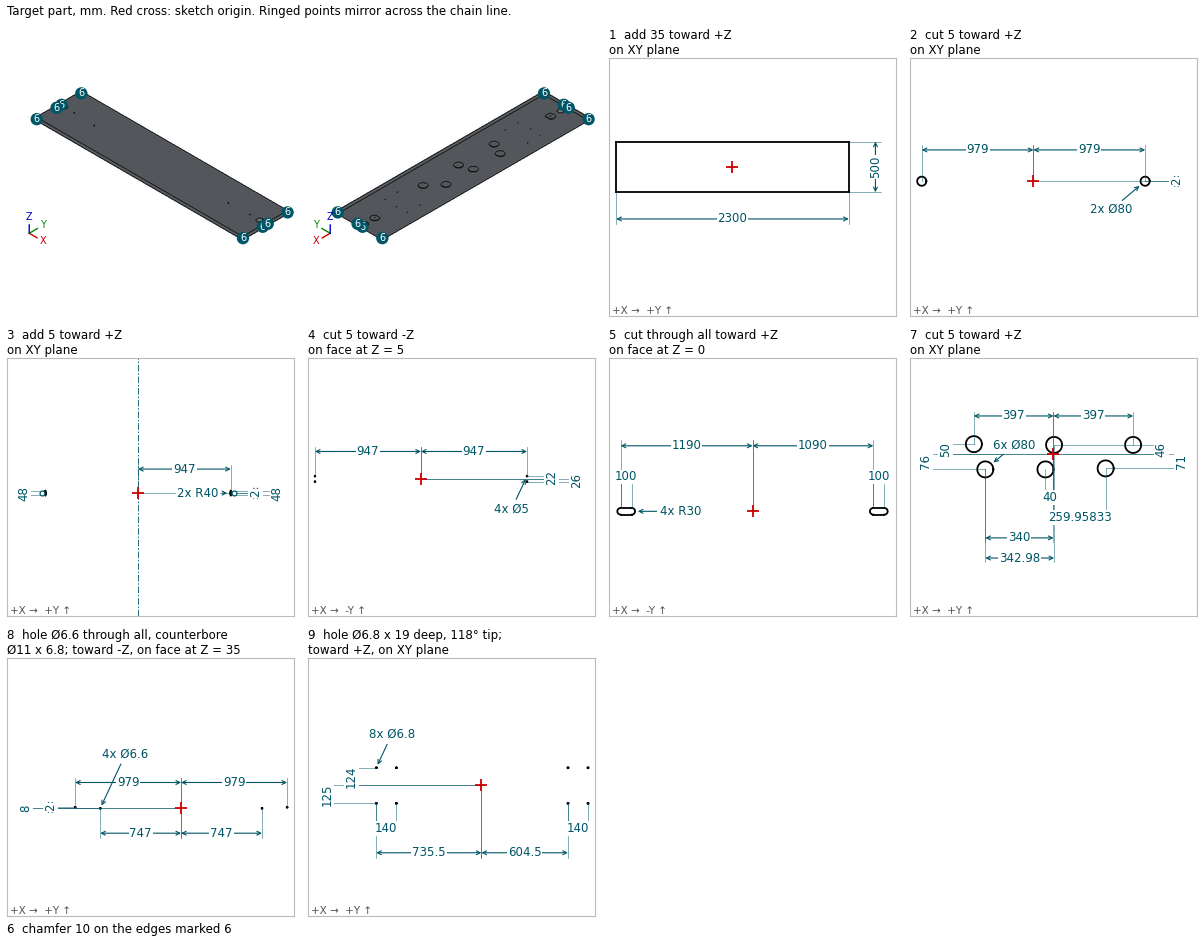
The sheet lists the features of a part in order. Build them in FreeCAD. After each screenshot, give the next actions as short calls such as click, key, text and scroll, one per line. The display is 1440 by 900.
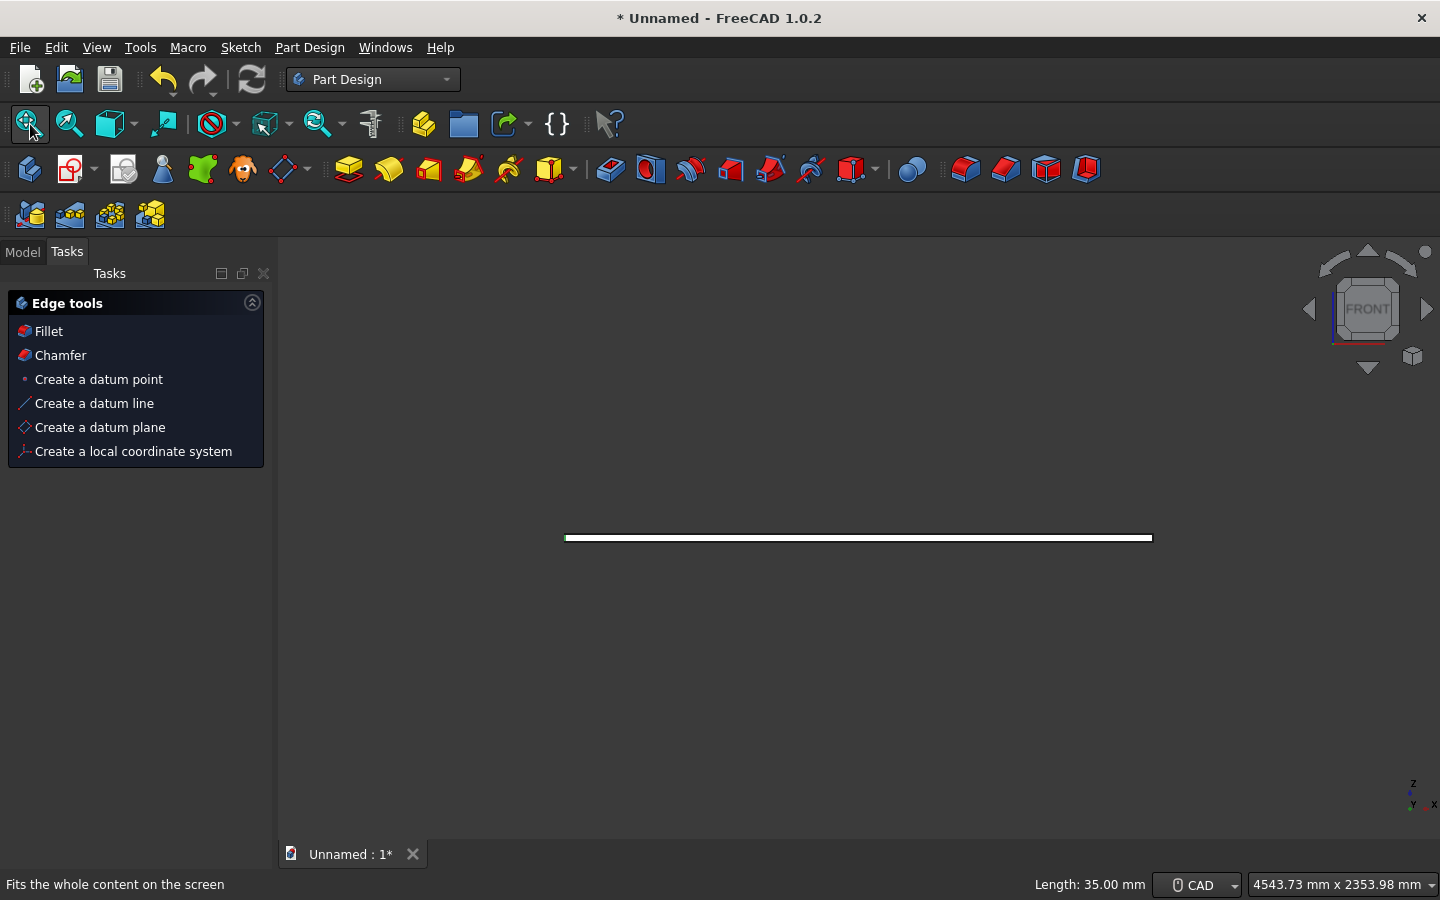
key(3)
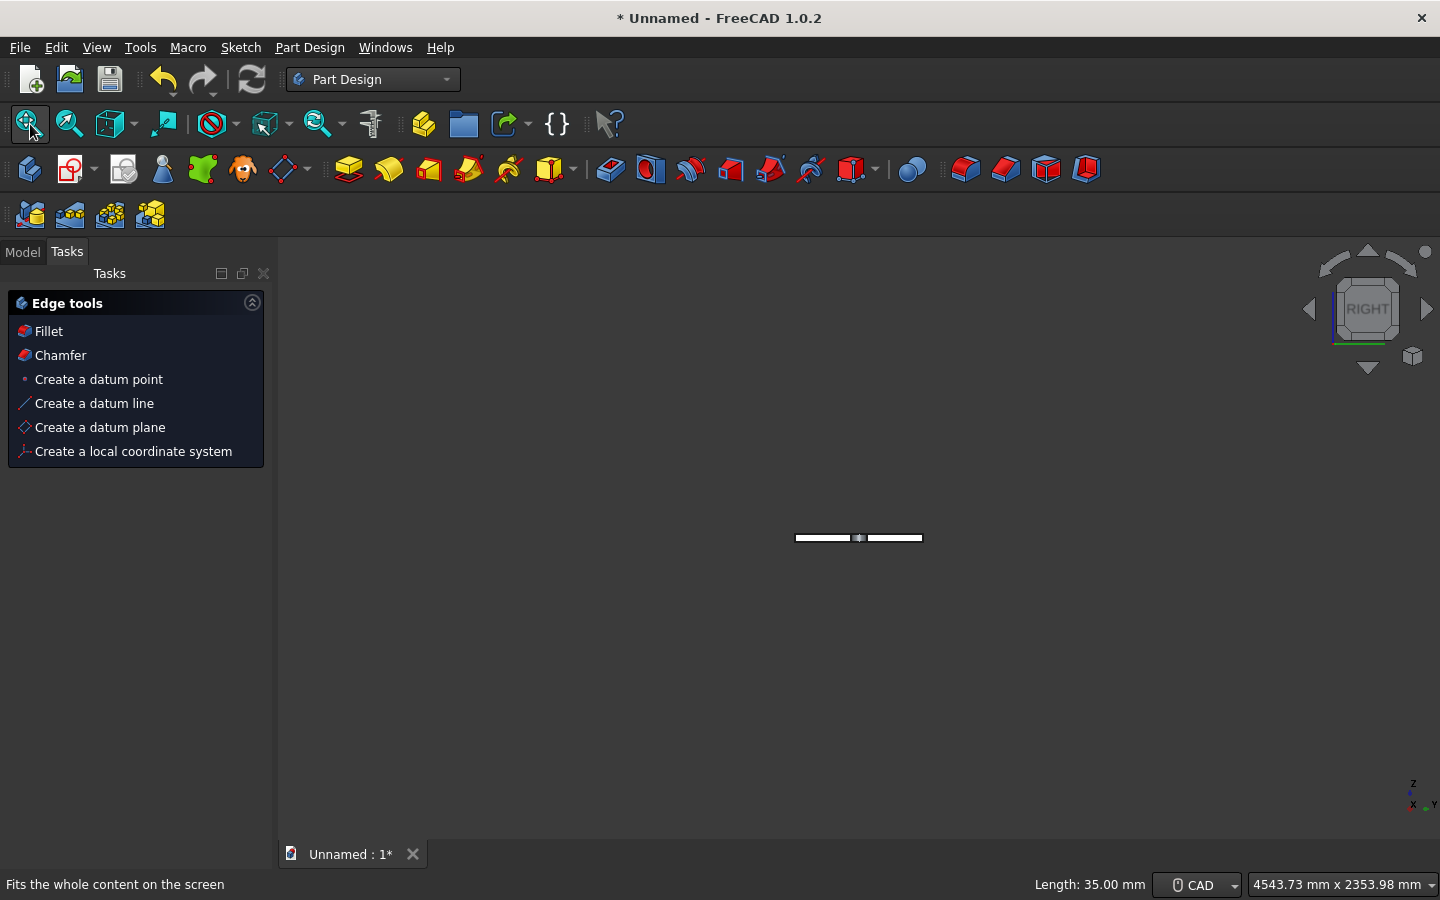
click(30, 124)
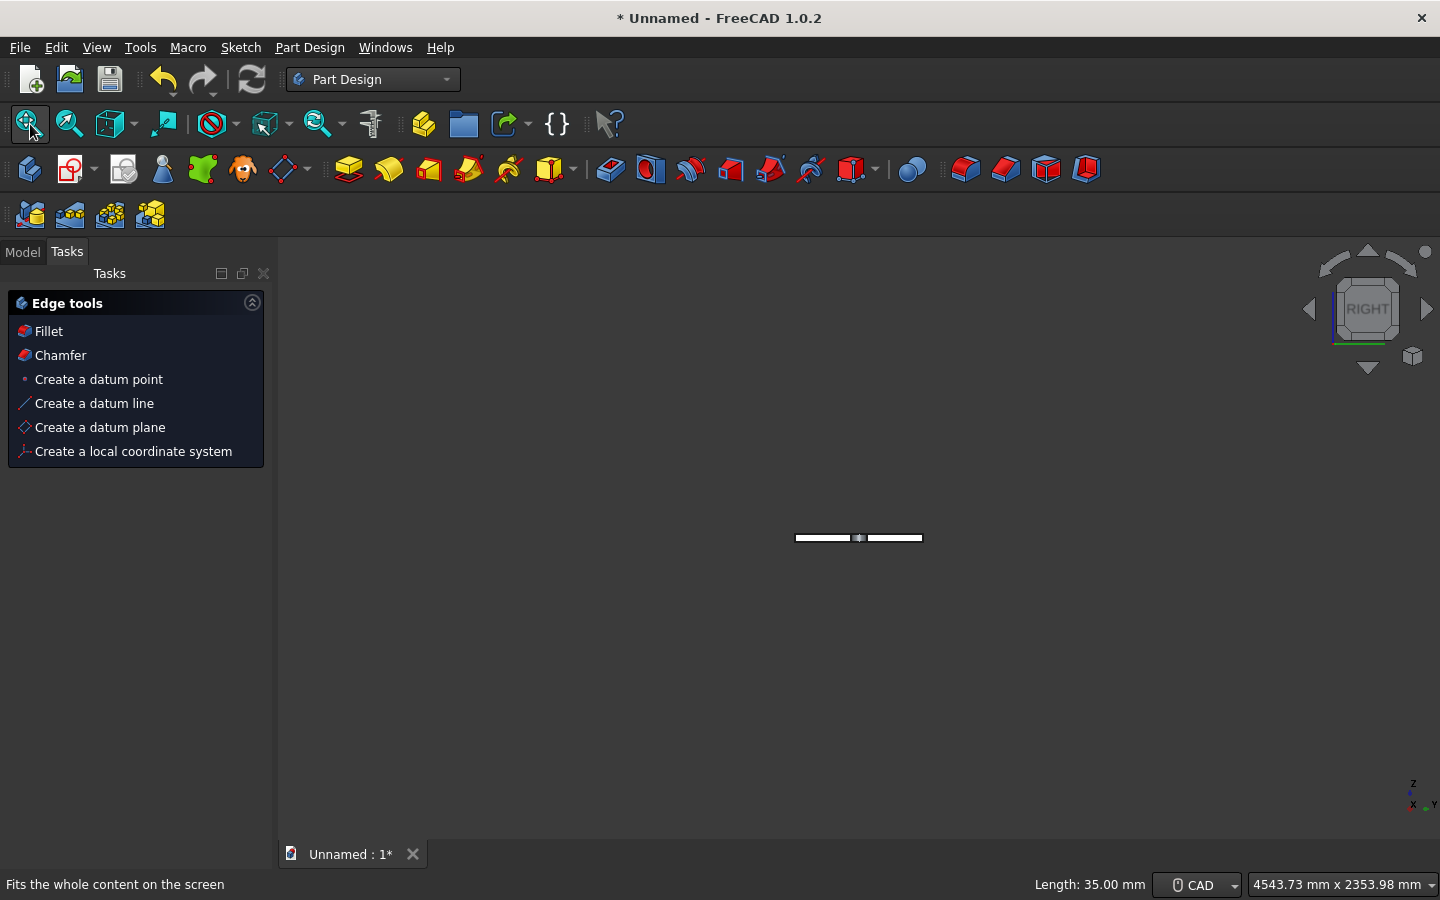
scroll(867, 537, up, 8)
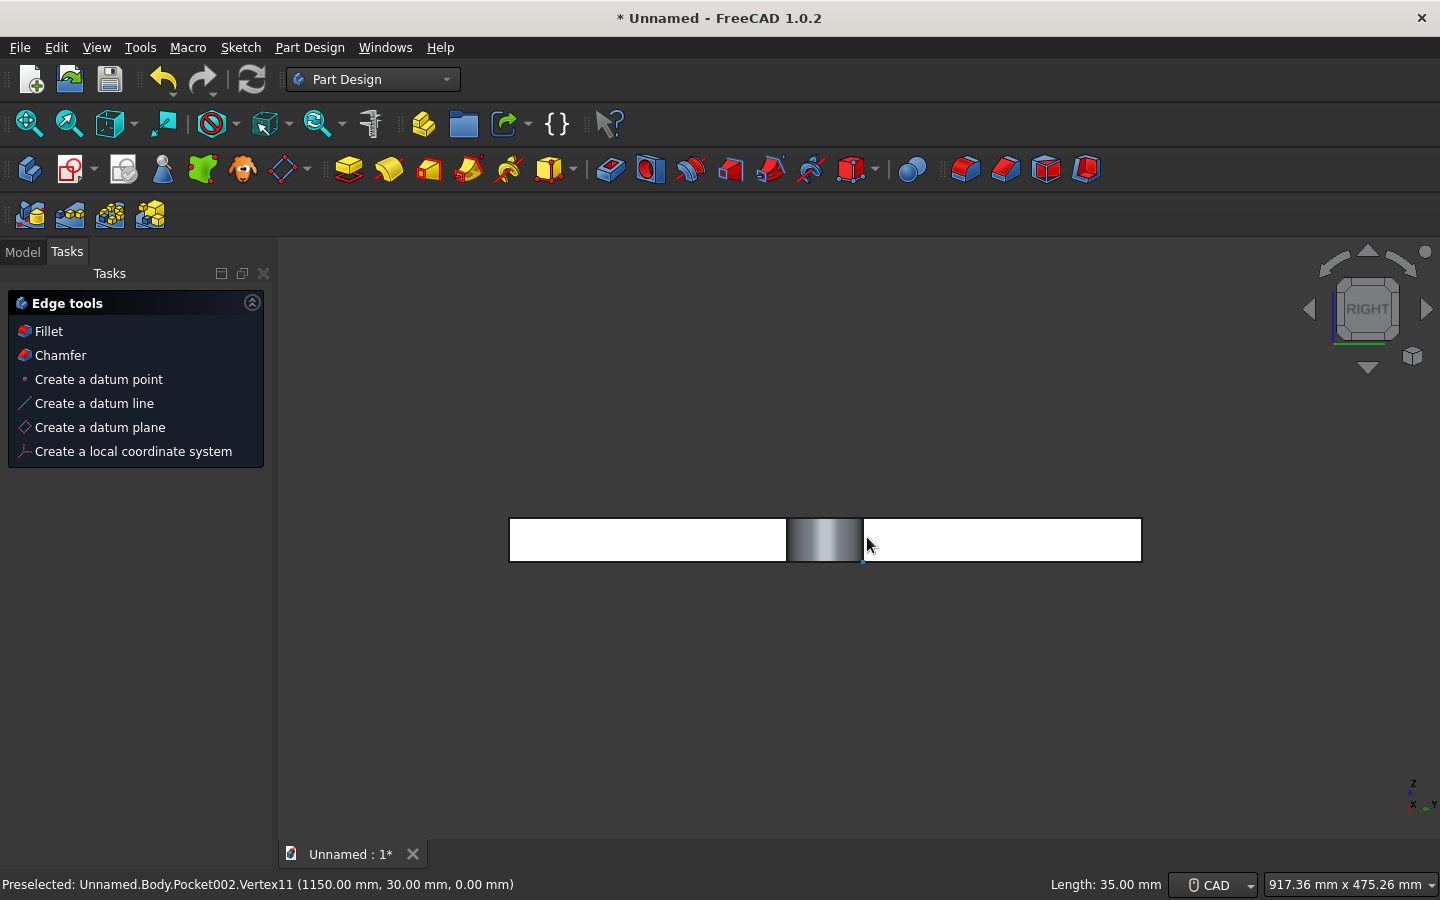
click(787, 539, ctrl)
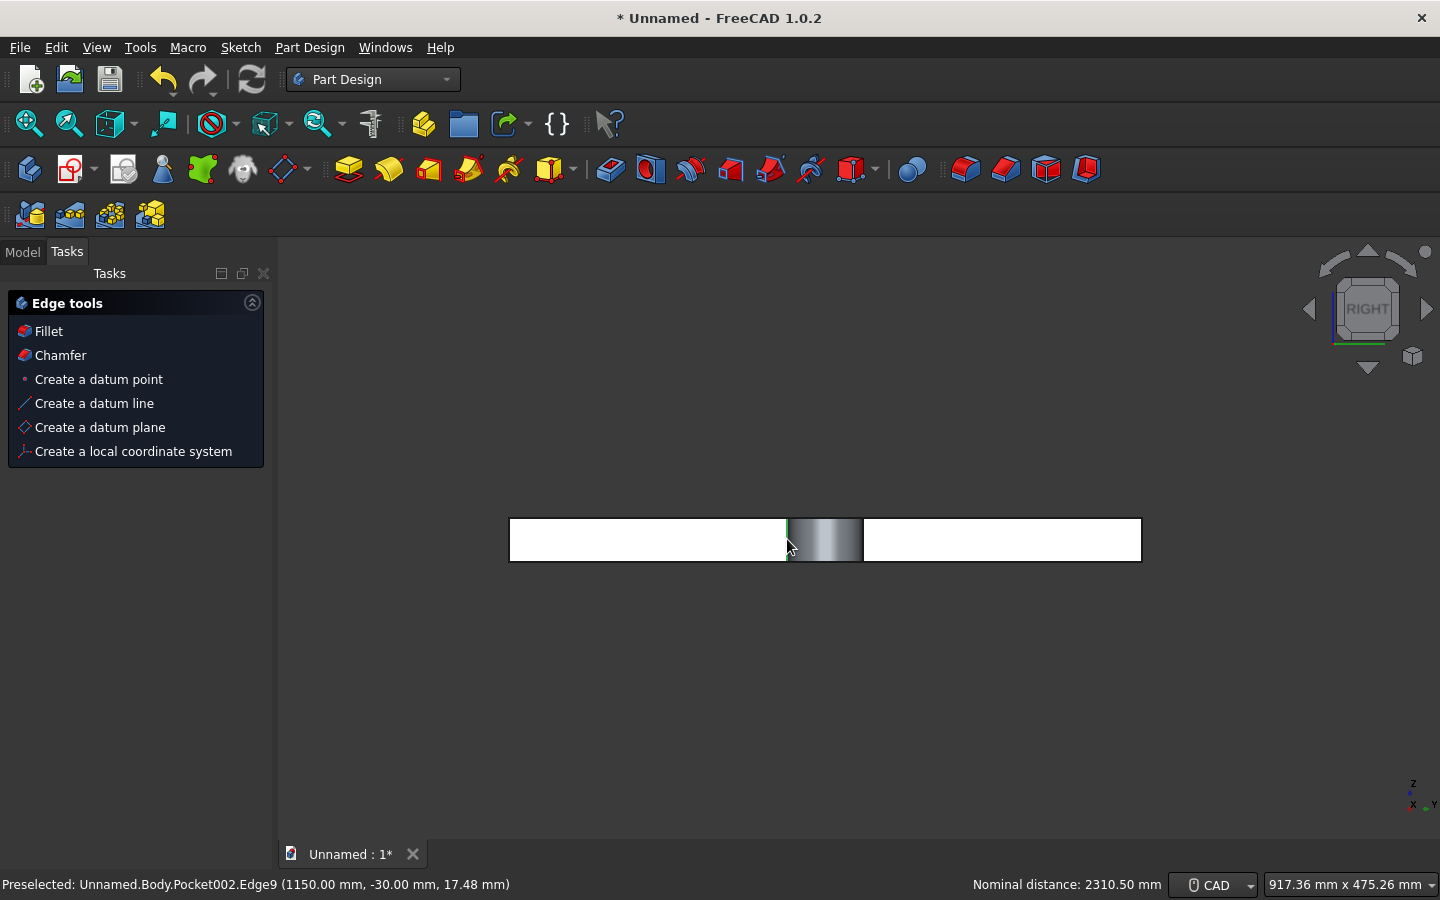
click(863, 539, ctrl)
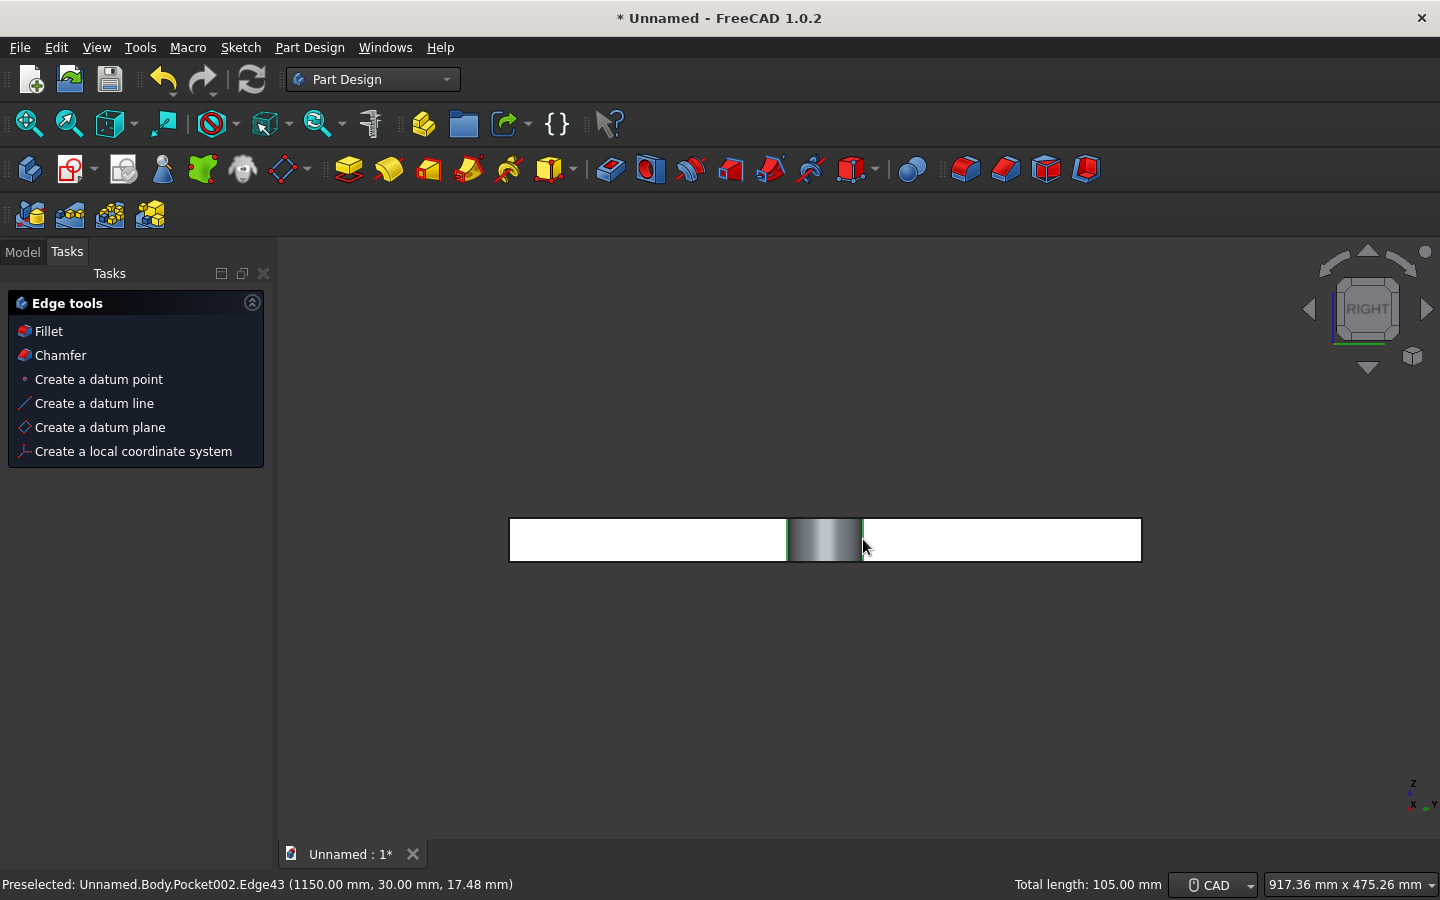
click(509, 539, ctrl)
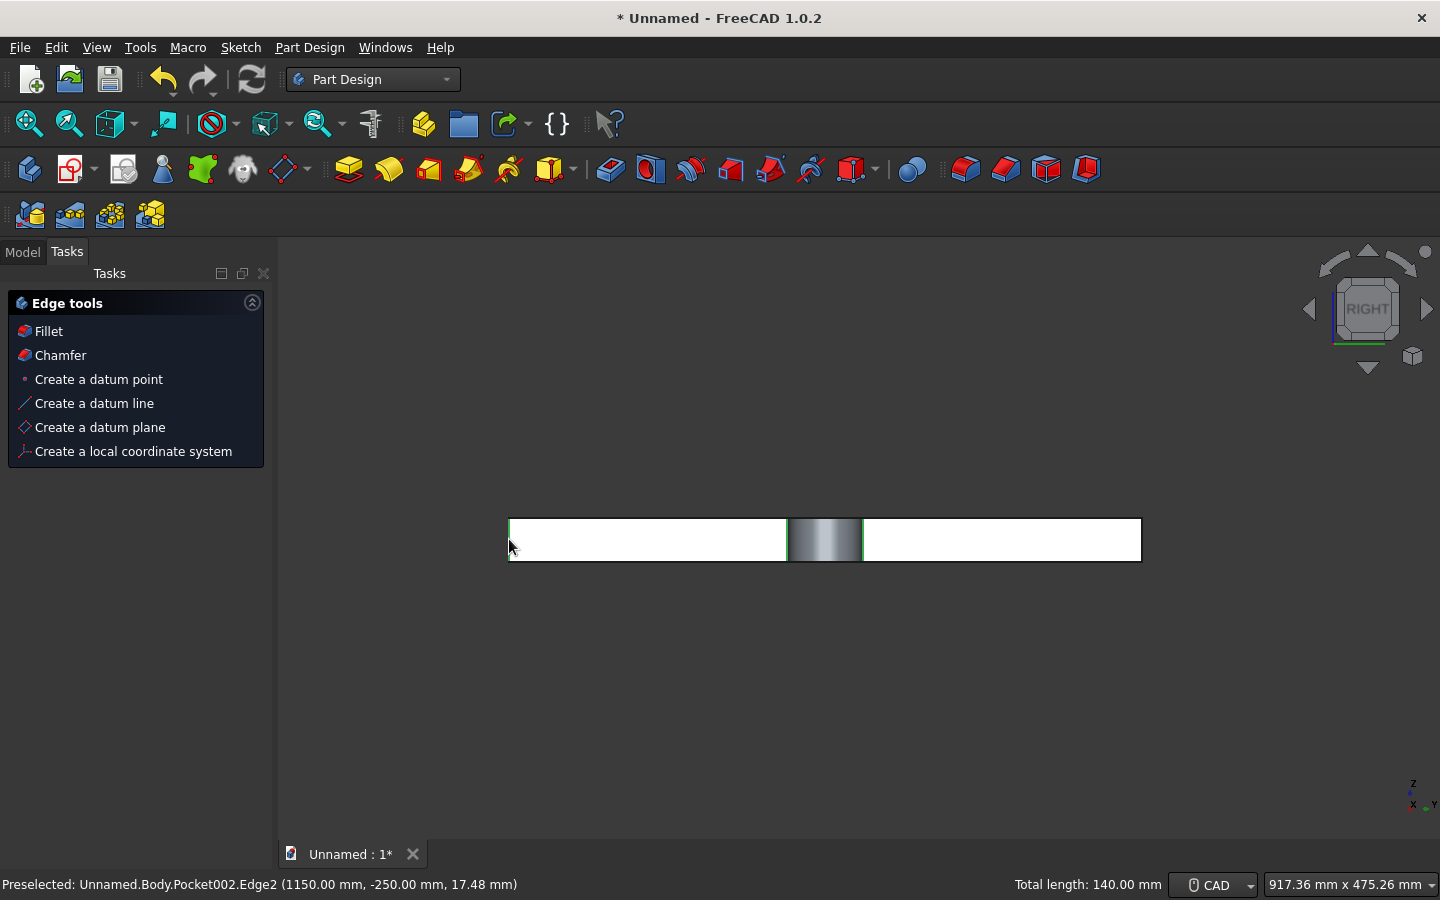
click(1142, 539, ctrl)